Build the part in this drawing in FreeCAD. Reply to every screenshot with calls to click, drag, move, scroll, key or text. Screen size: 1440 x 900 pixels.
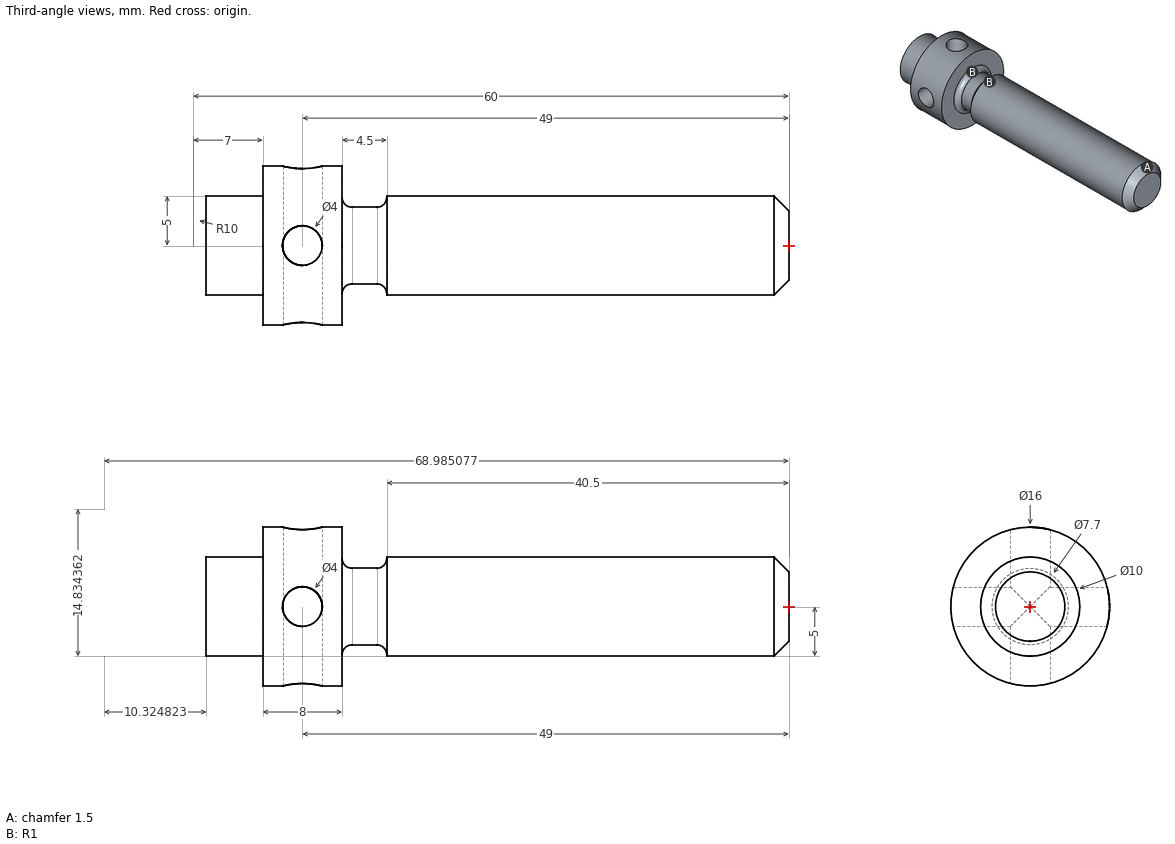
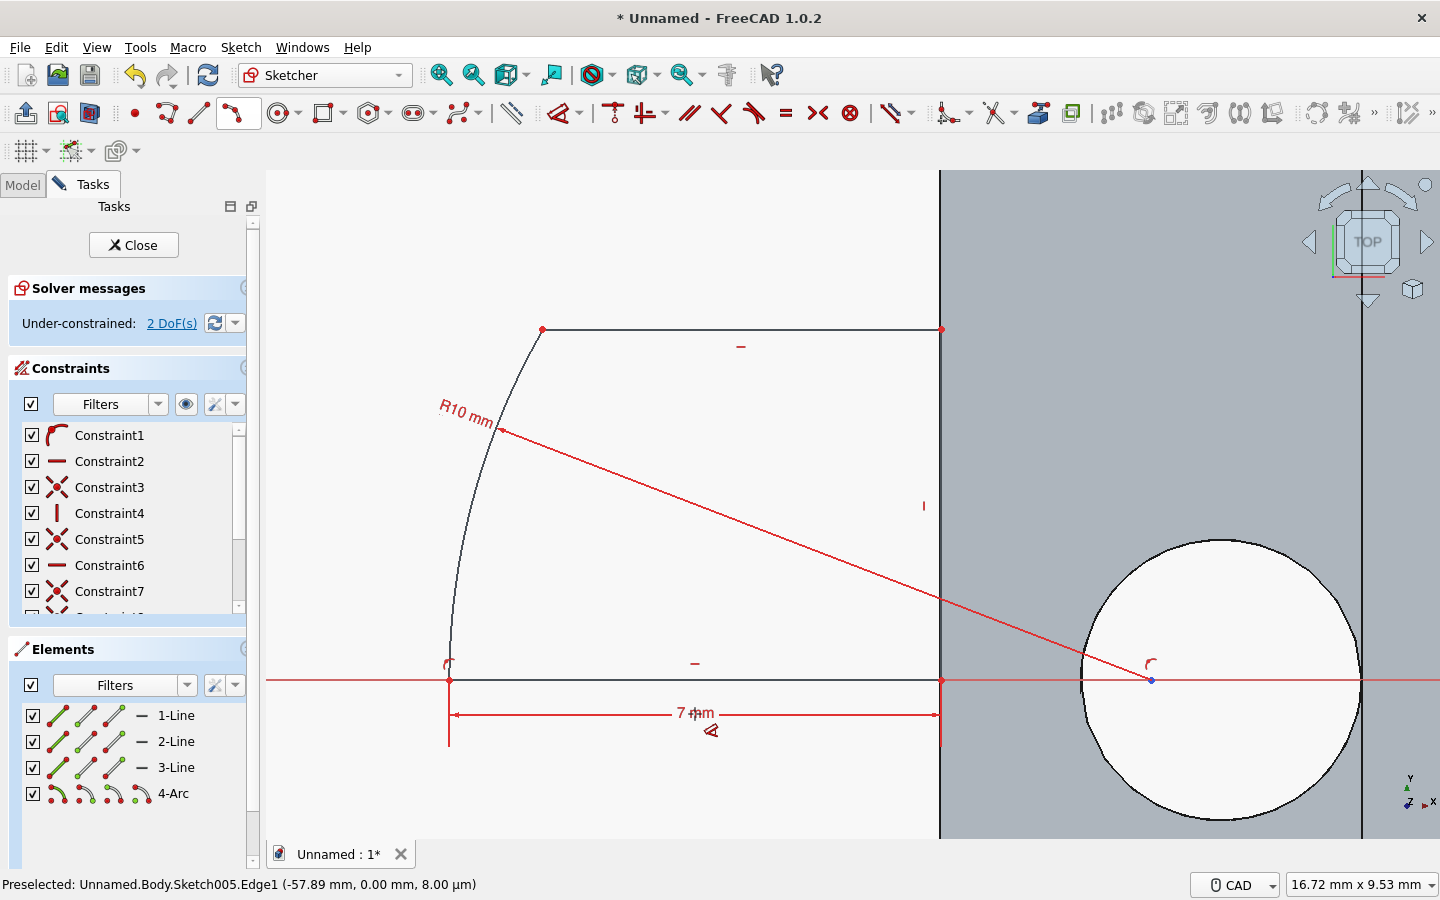
click(941, 575)
click(975, 505)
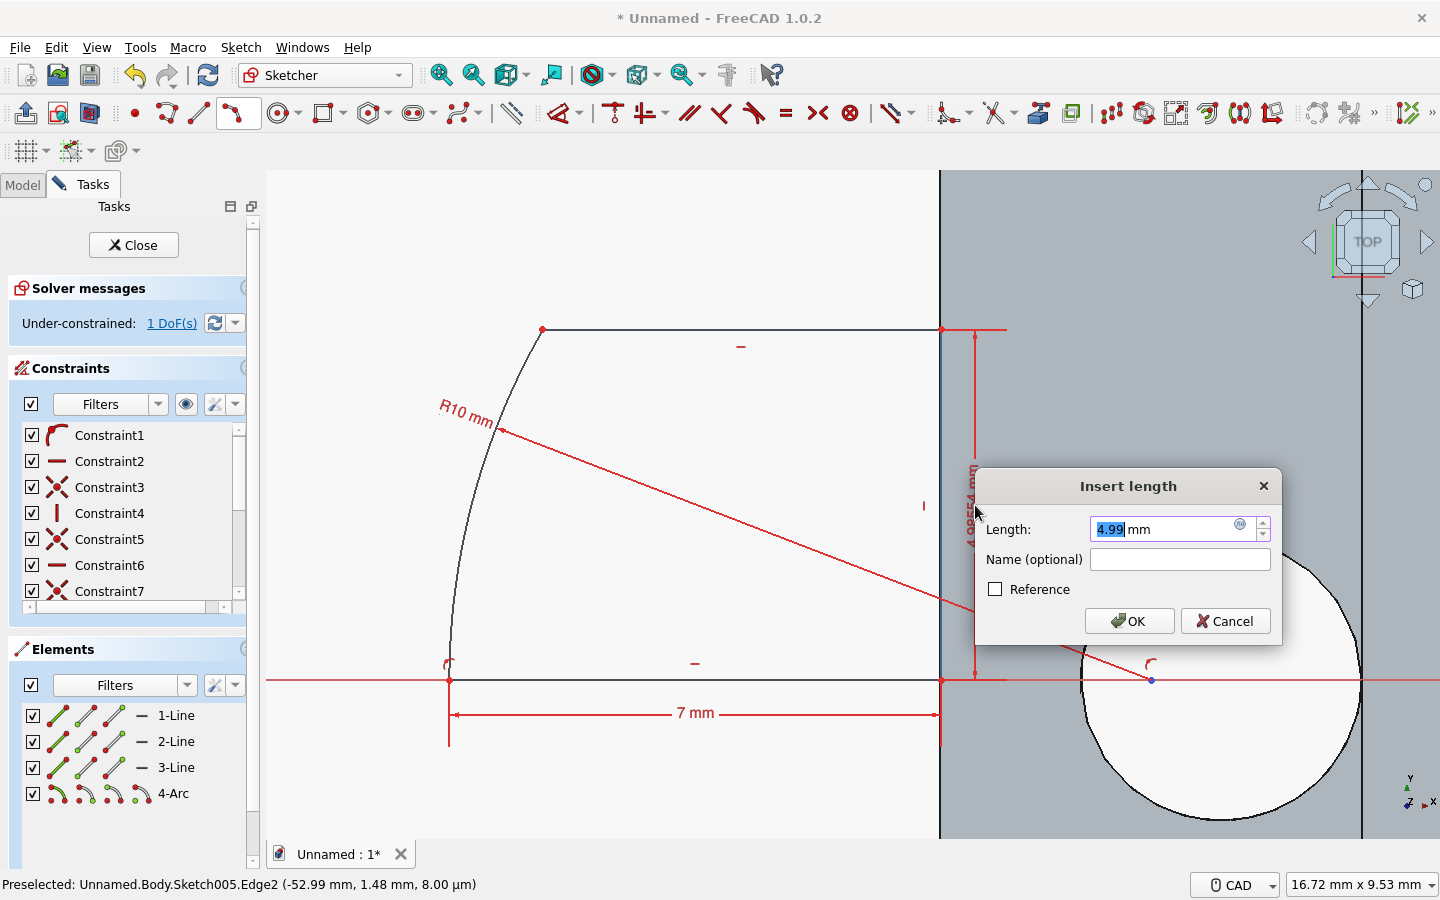
text(5)
key(Return)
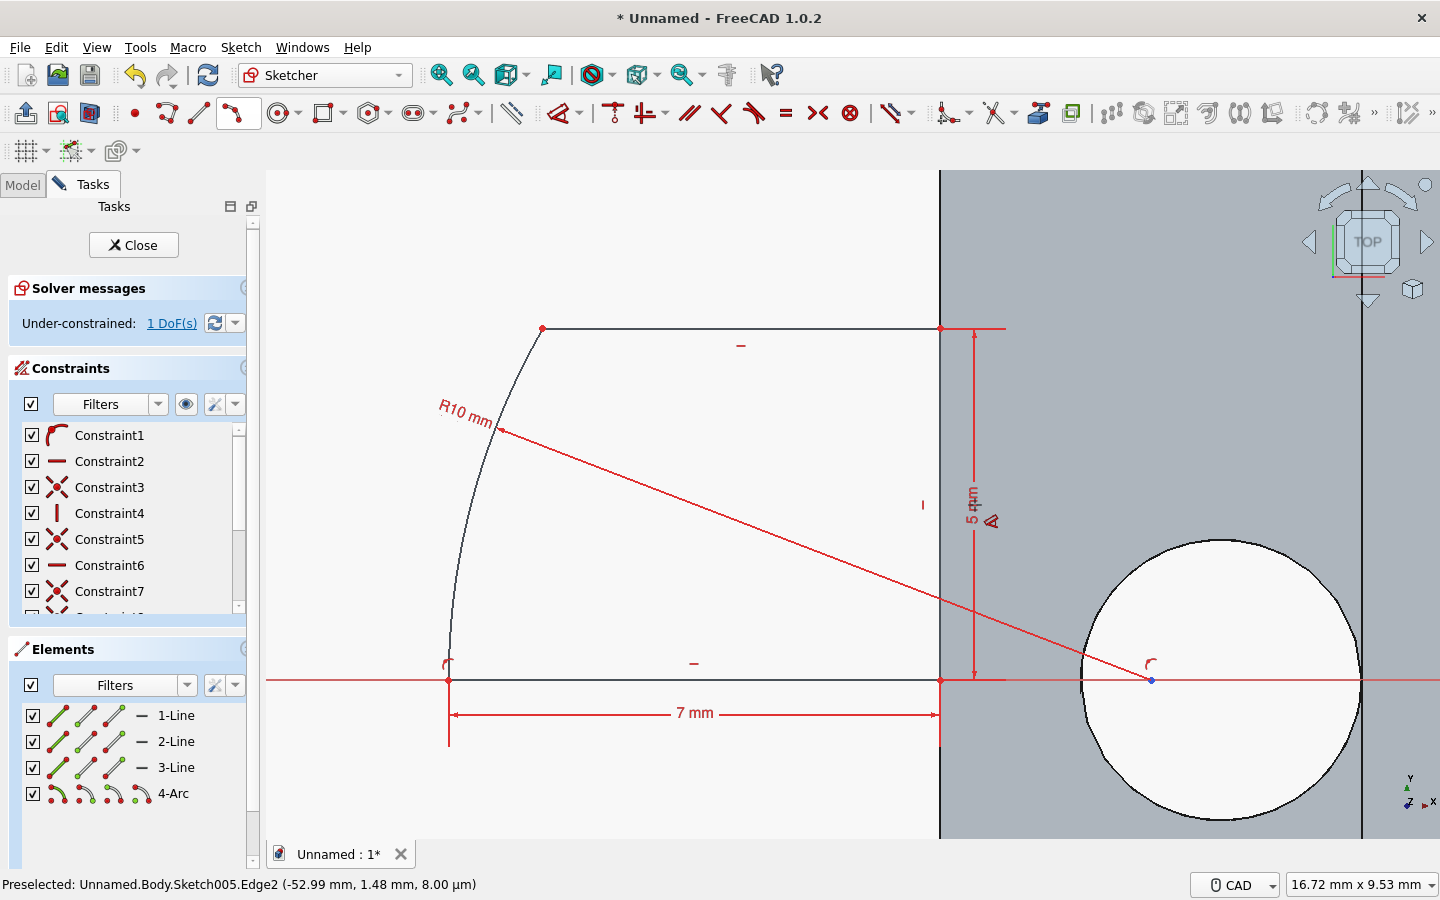
click(449, 680)
click(862, 714)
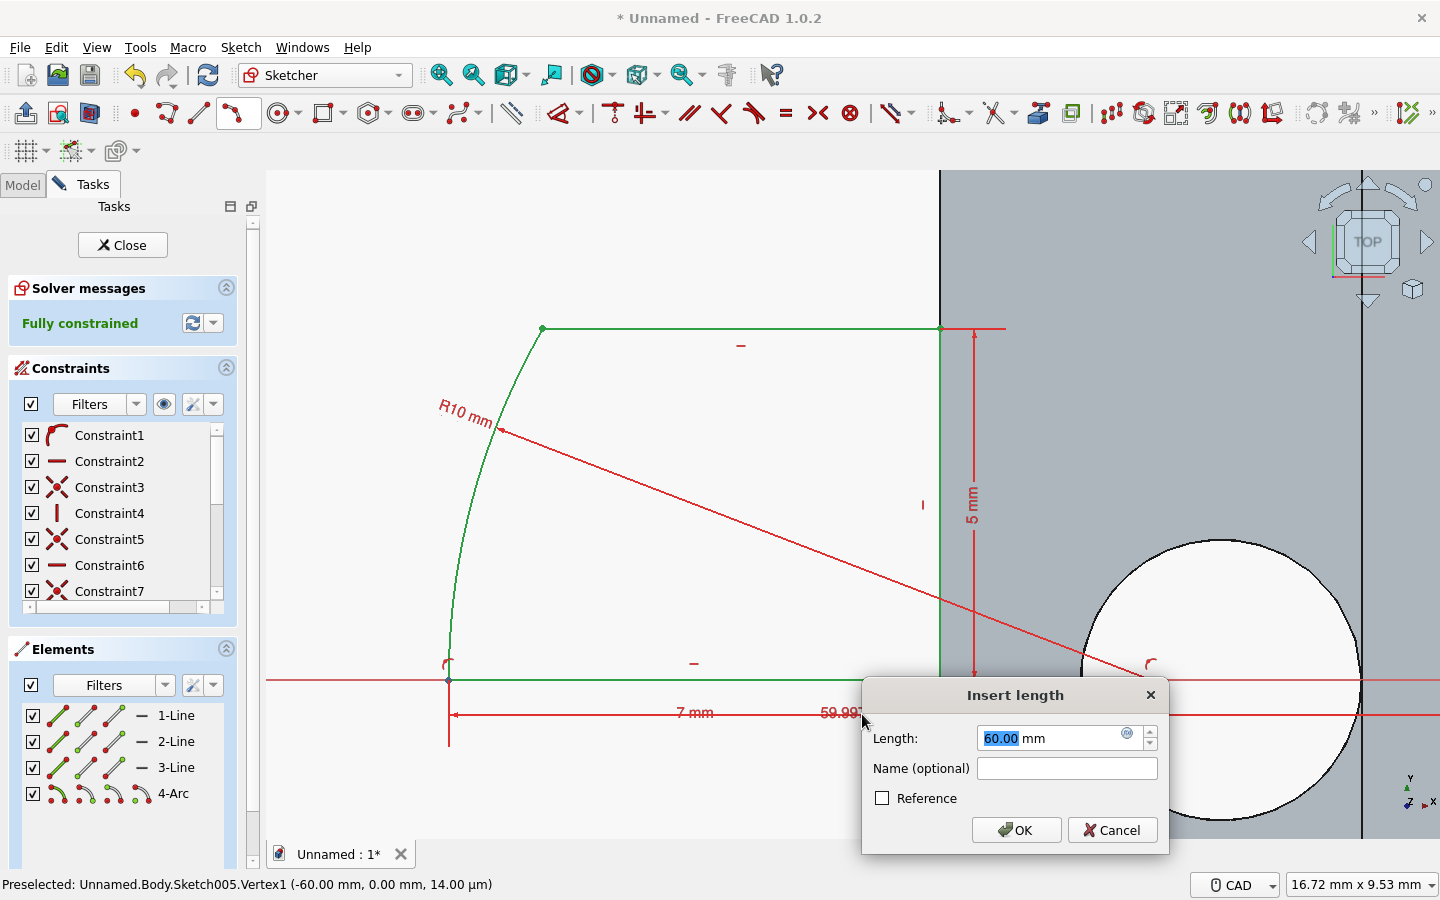
text(60)
key(Return)
key(Escape)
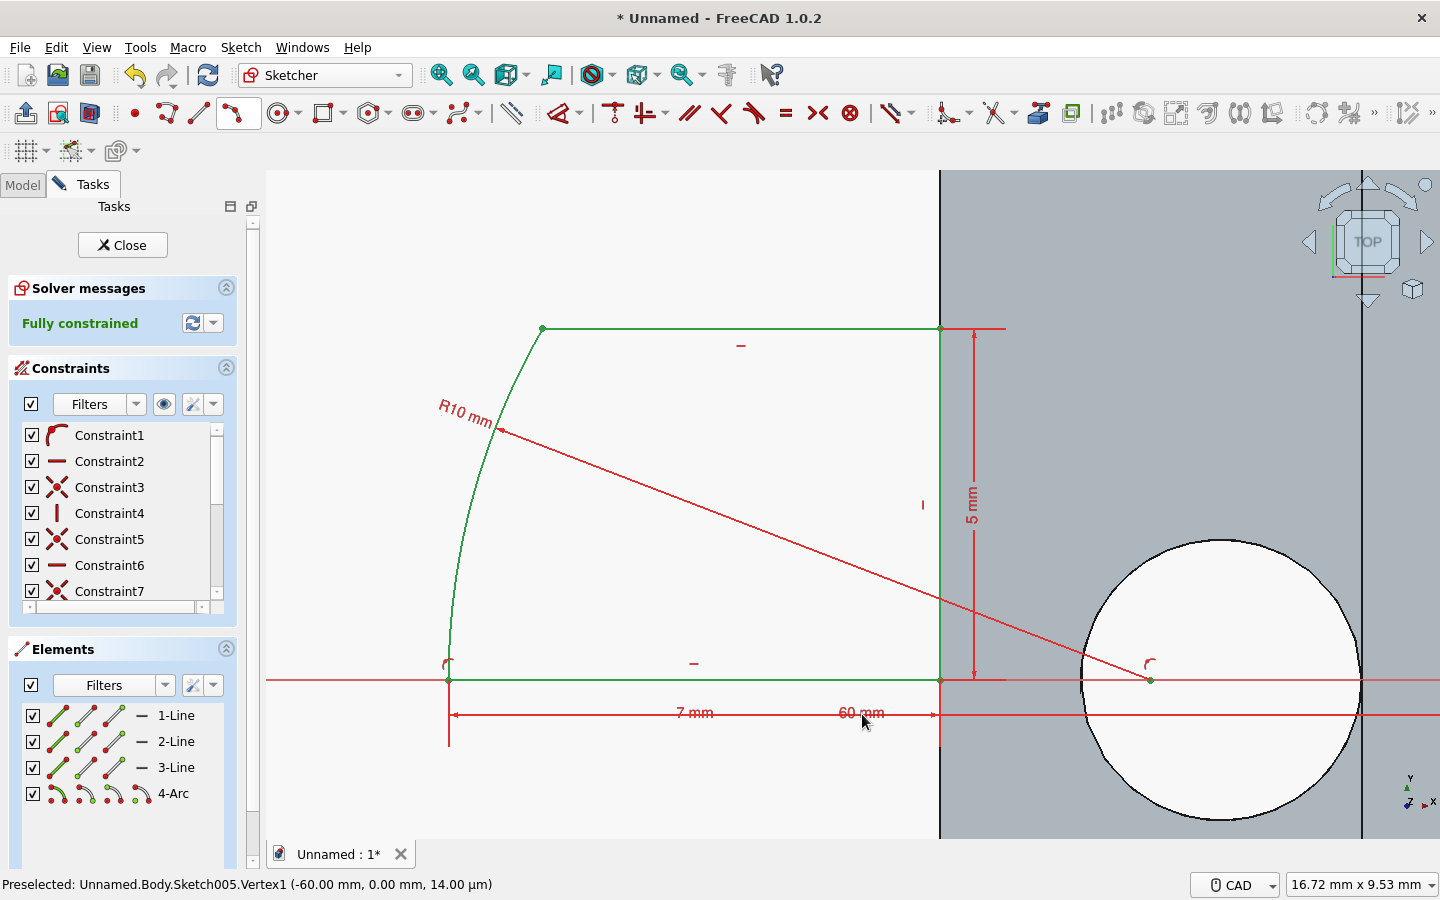
click(123, 245)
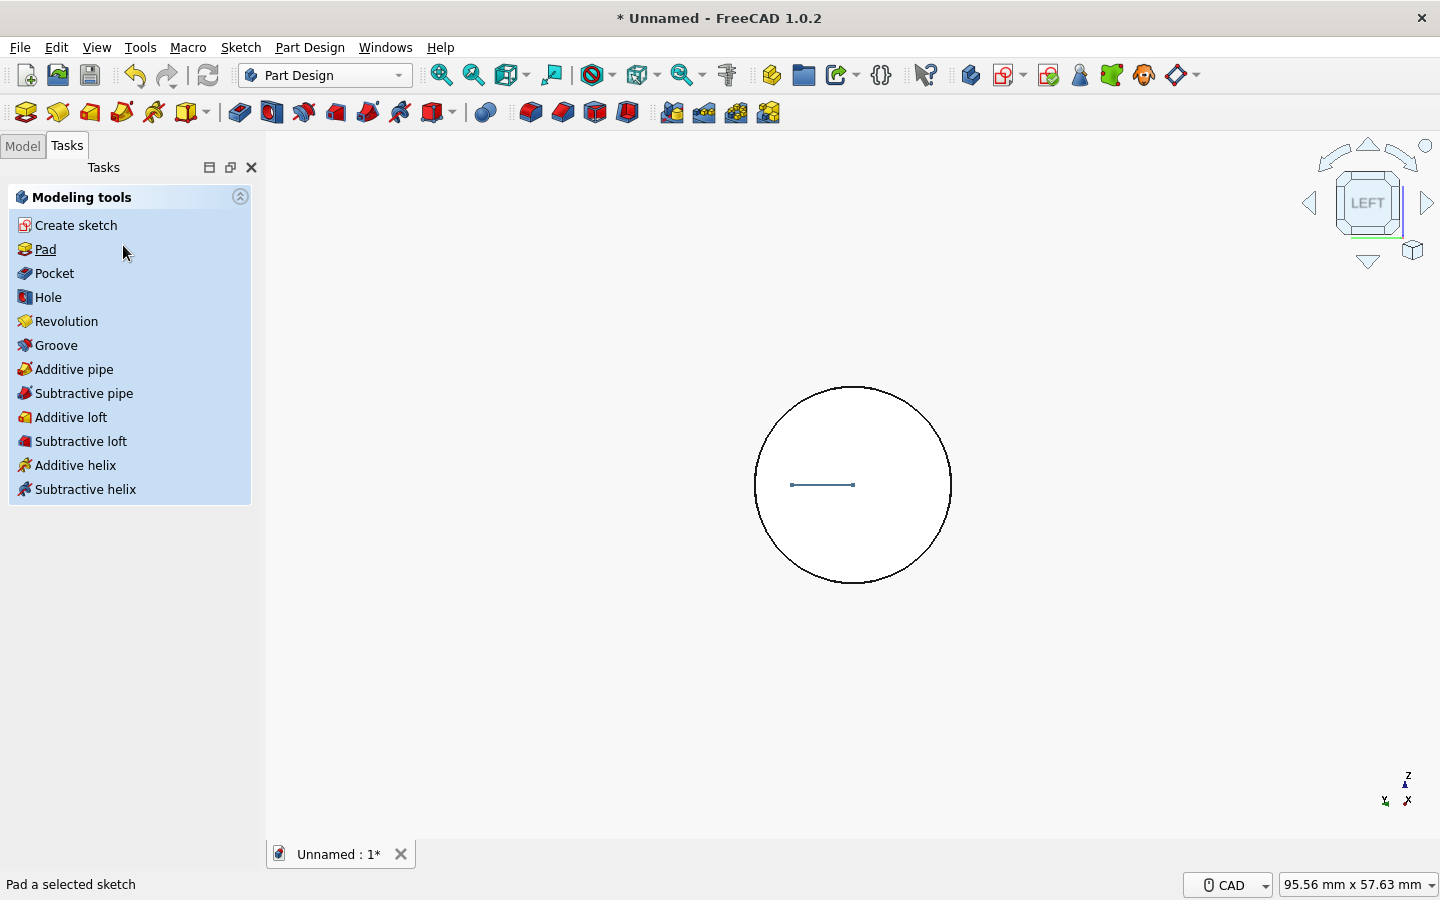
click(58, 112)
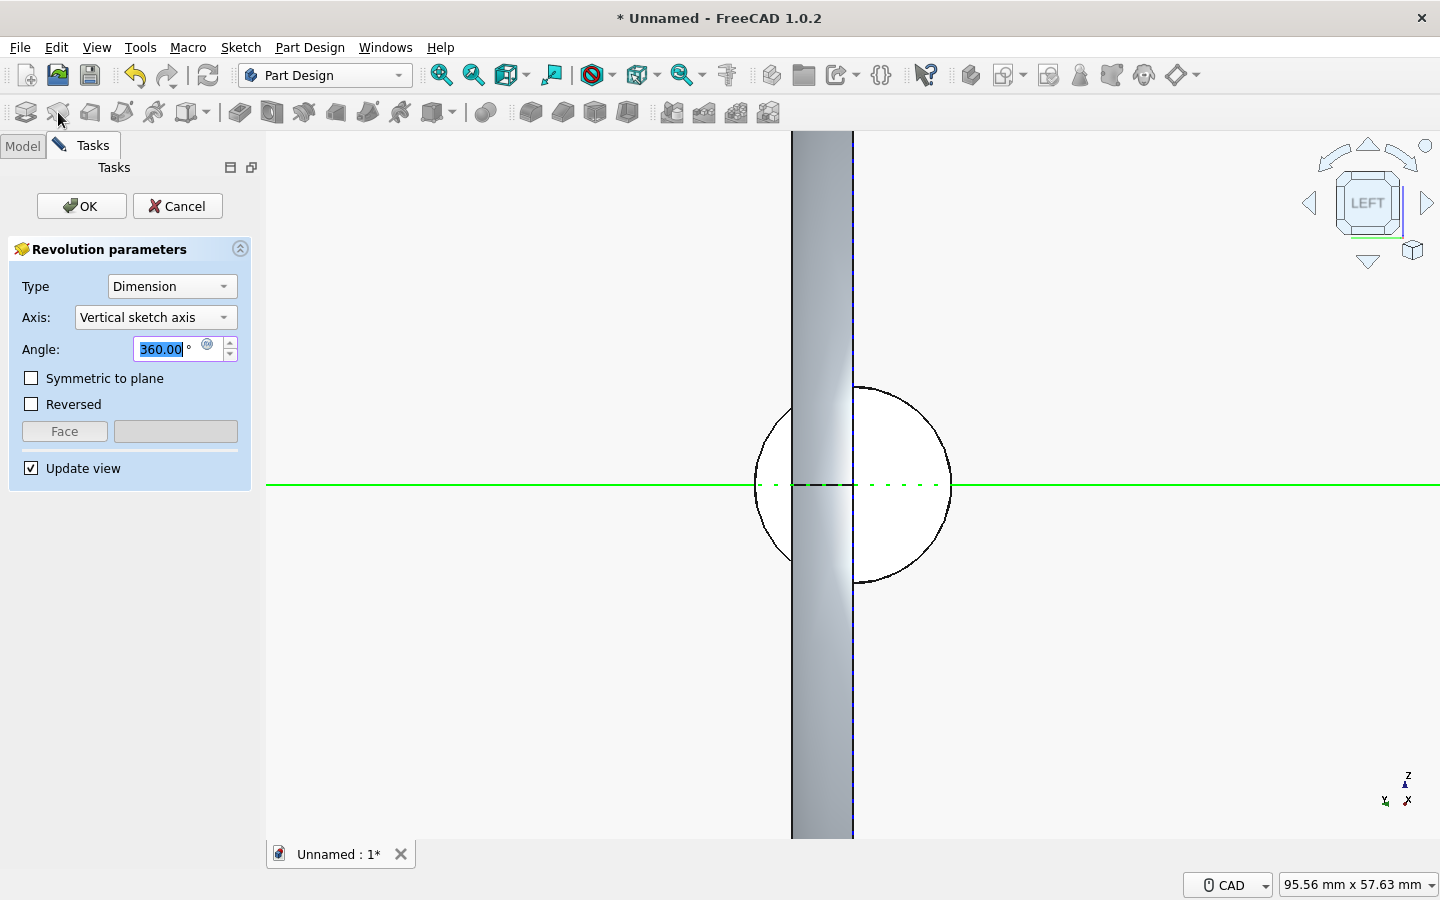
click(156, 318)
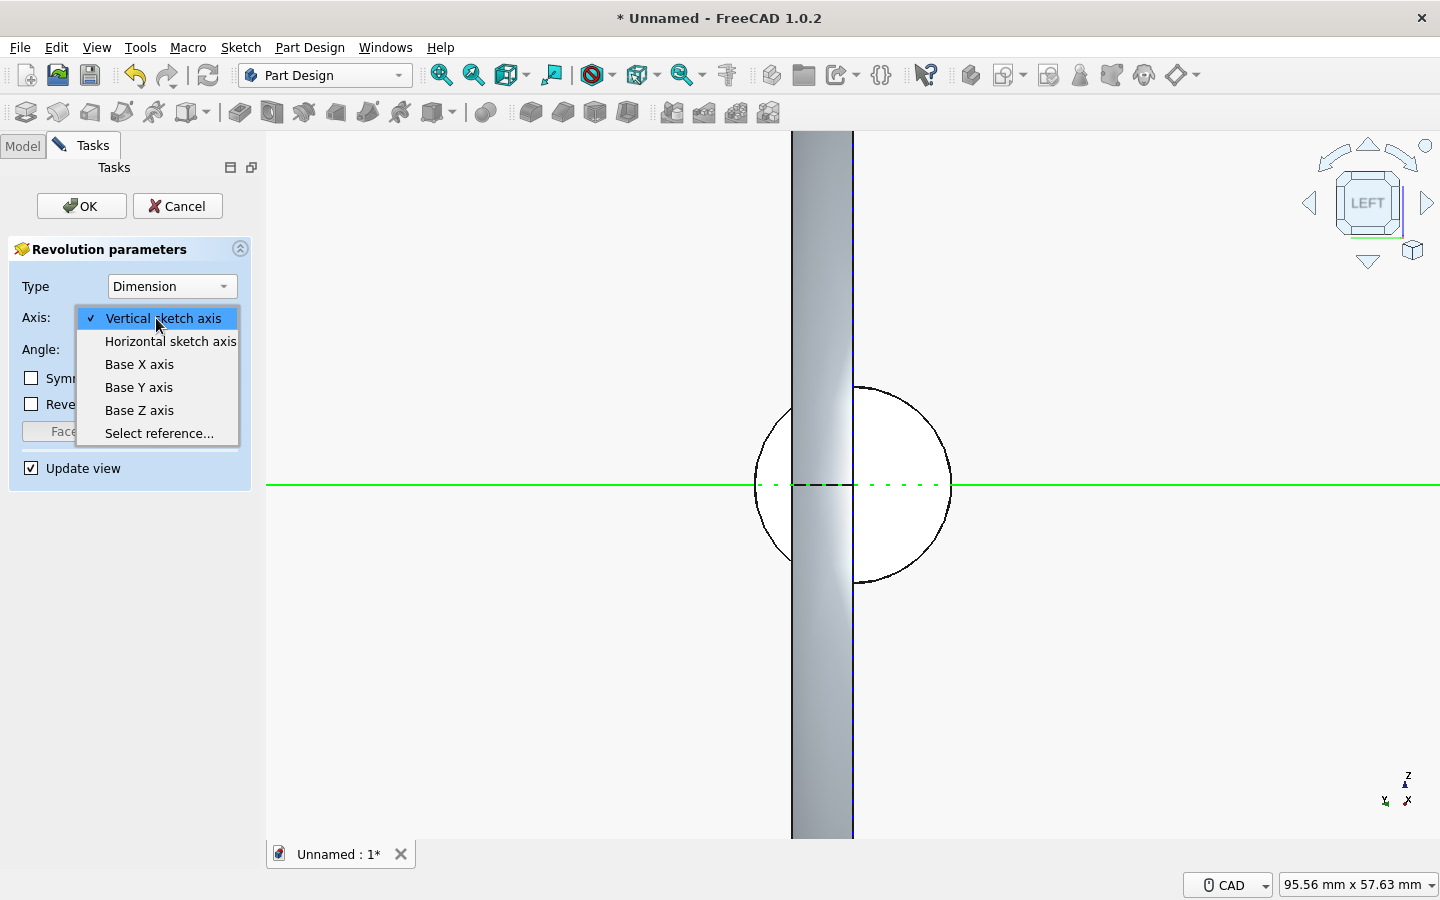
click(156, 342)